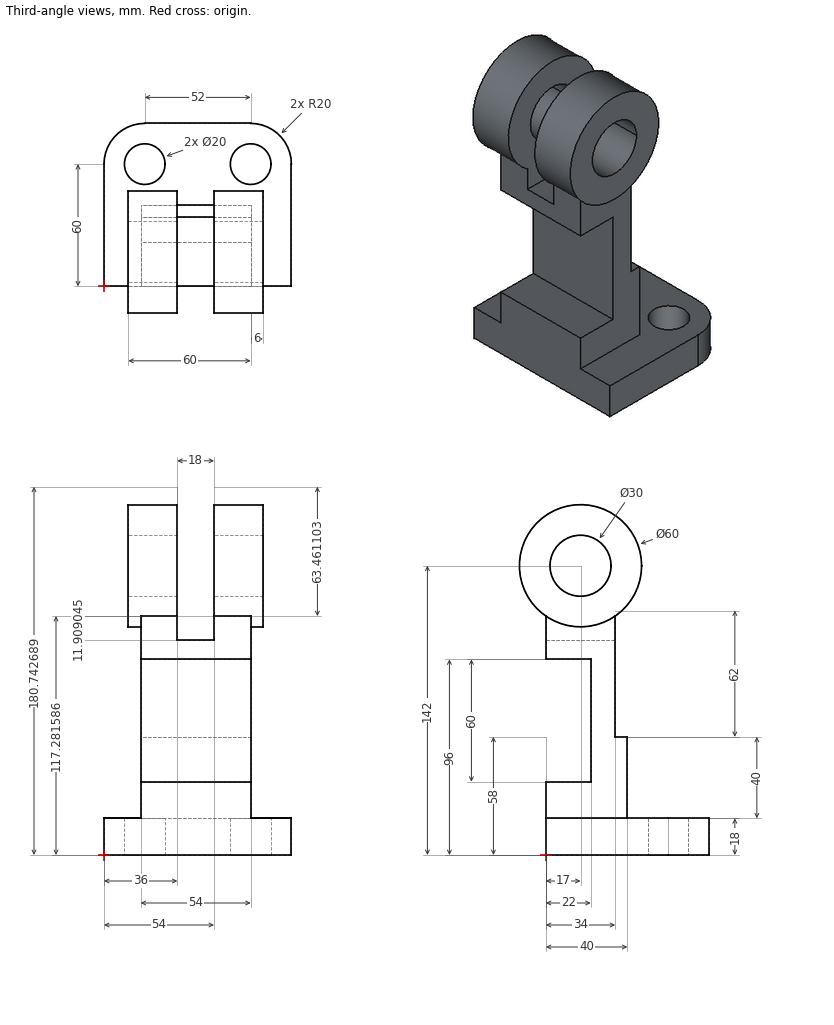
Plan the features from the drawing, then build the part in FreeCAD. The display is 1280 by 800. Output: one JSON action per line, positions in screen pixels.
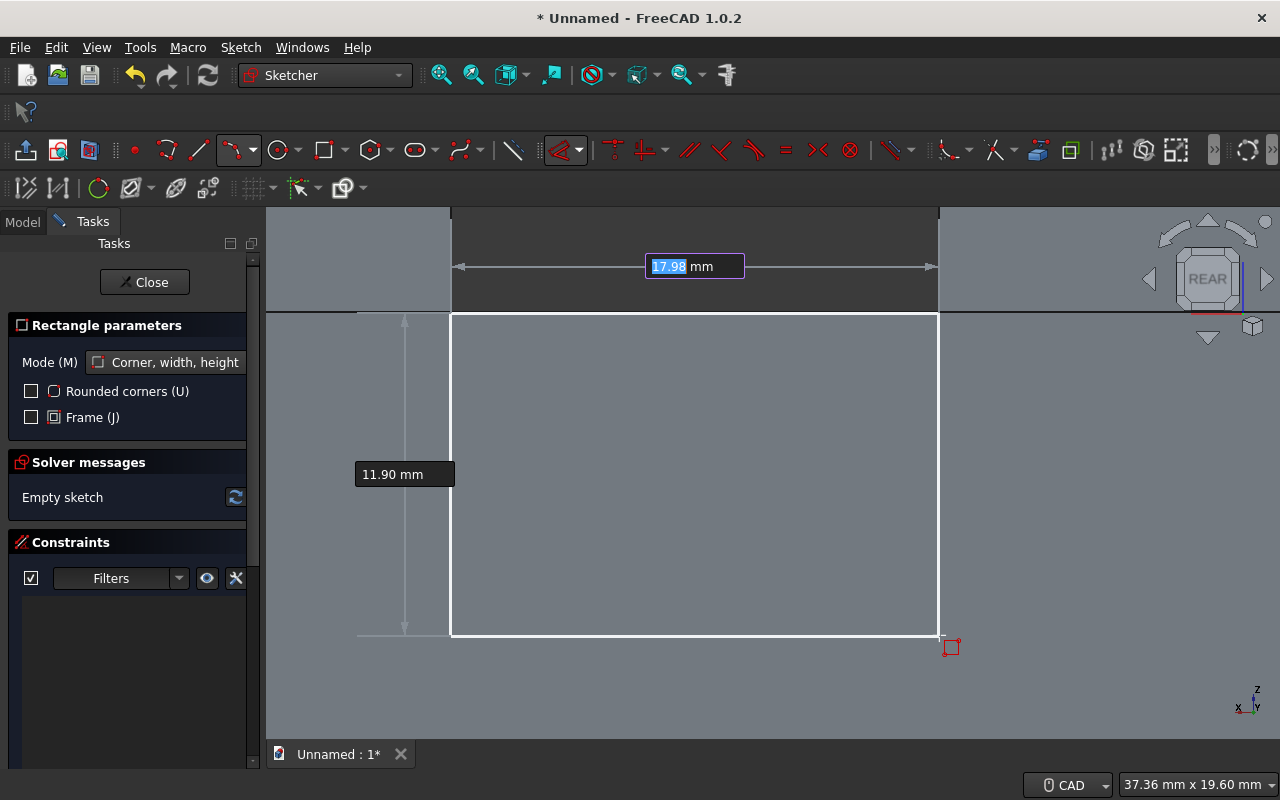
{"action": "type", "text": "18"}
{"action": "key", "text": "Tab"}
{"action": "type", "text": "11.909045"}
{"action": "key", "text": "Return"}
{"action": "key", "text": "Escape"}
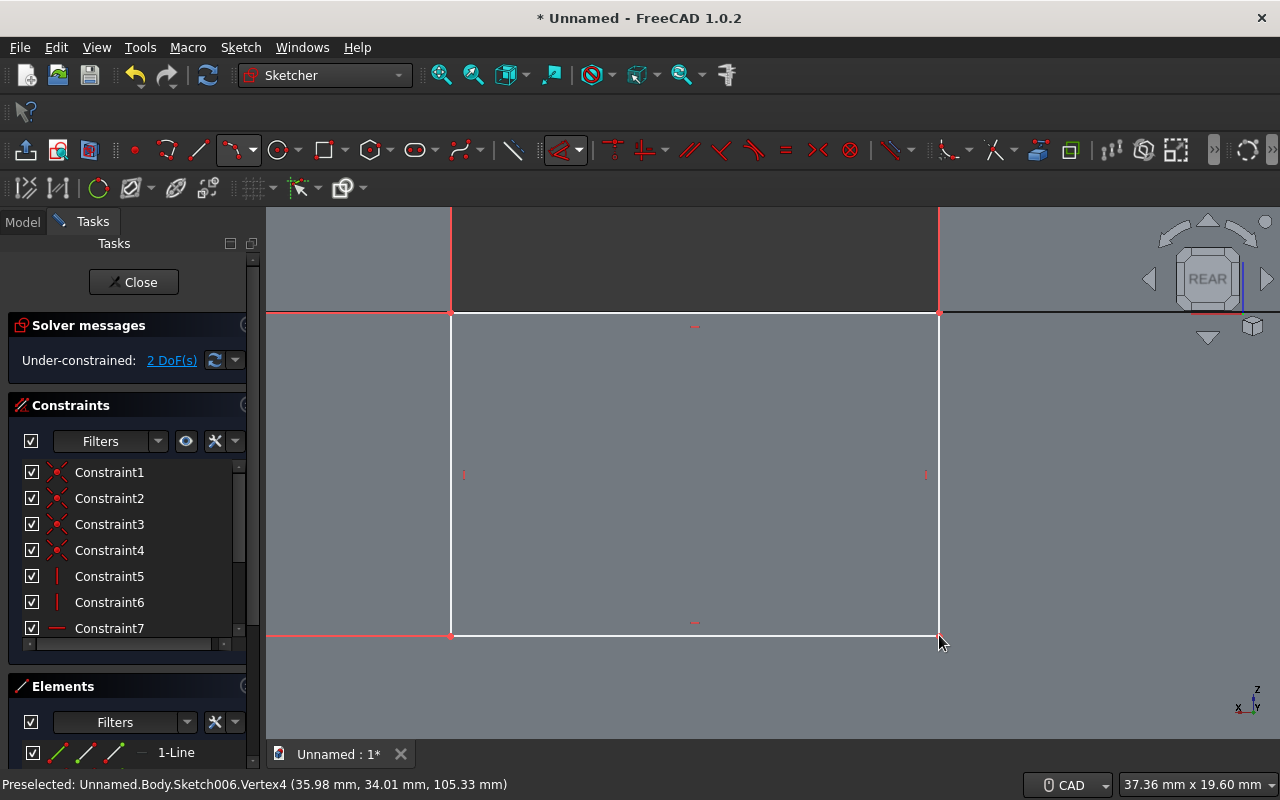
{"action": "left_click", "coordinate": [451, 313]}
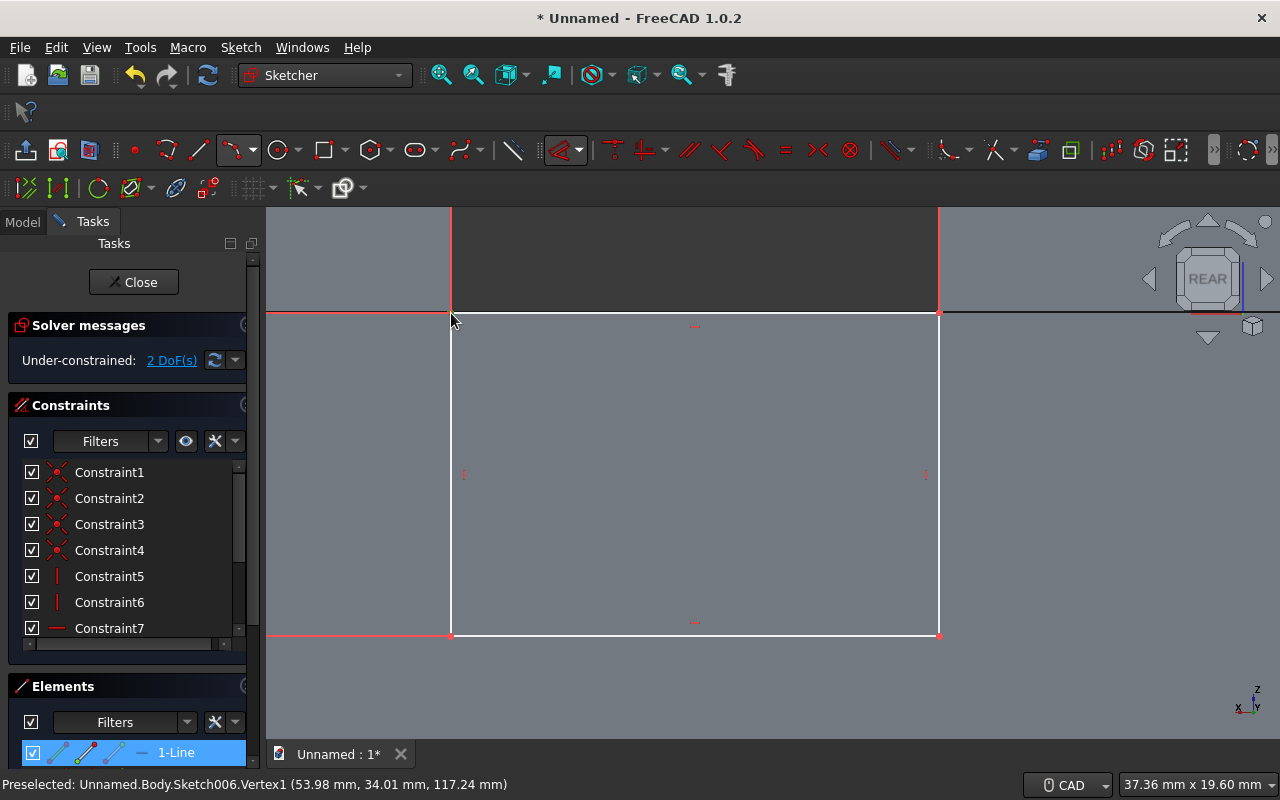
{"action": "left_click", "coordinate": [582, 150]}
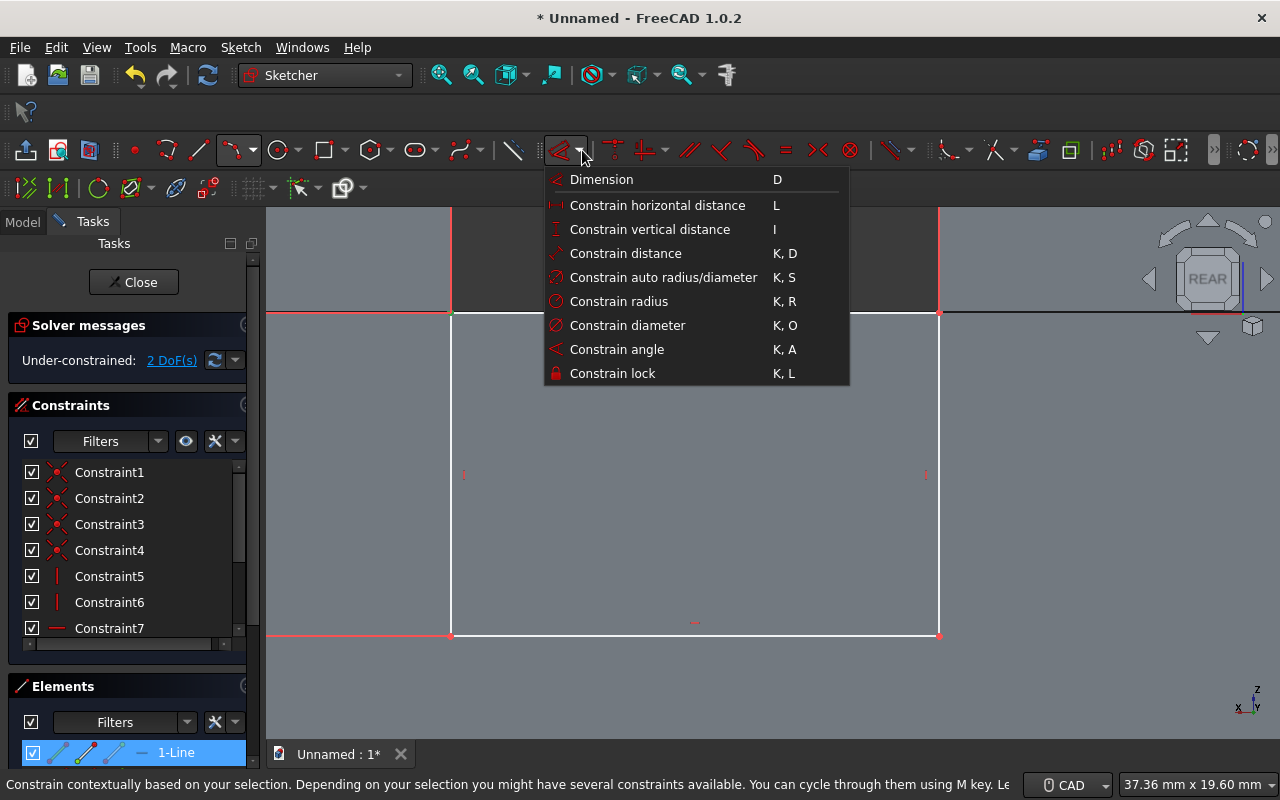
{"action": "left_click", "coordinate": [697, 205]}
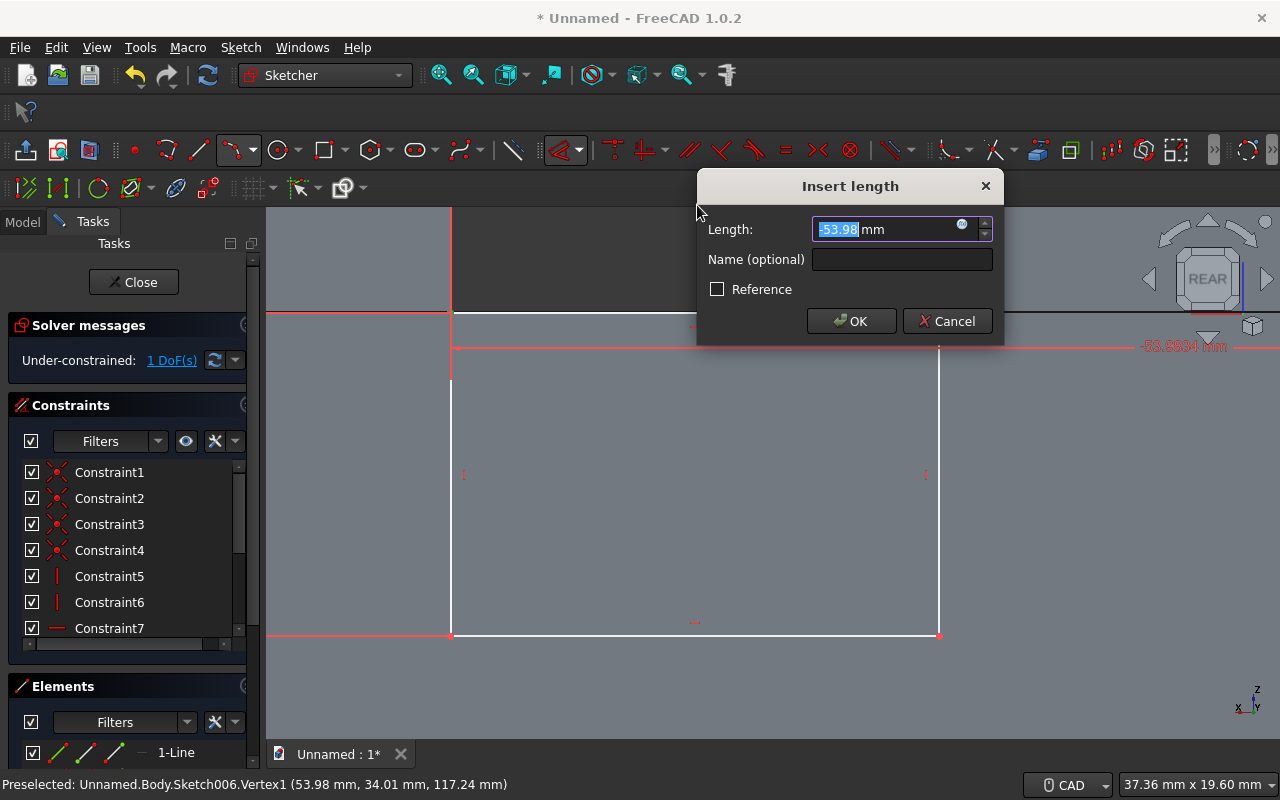
{"action": "type", "text": "-54"}
{"action": "key", "text": "Return"}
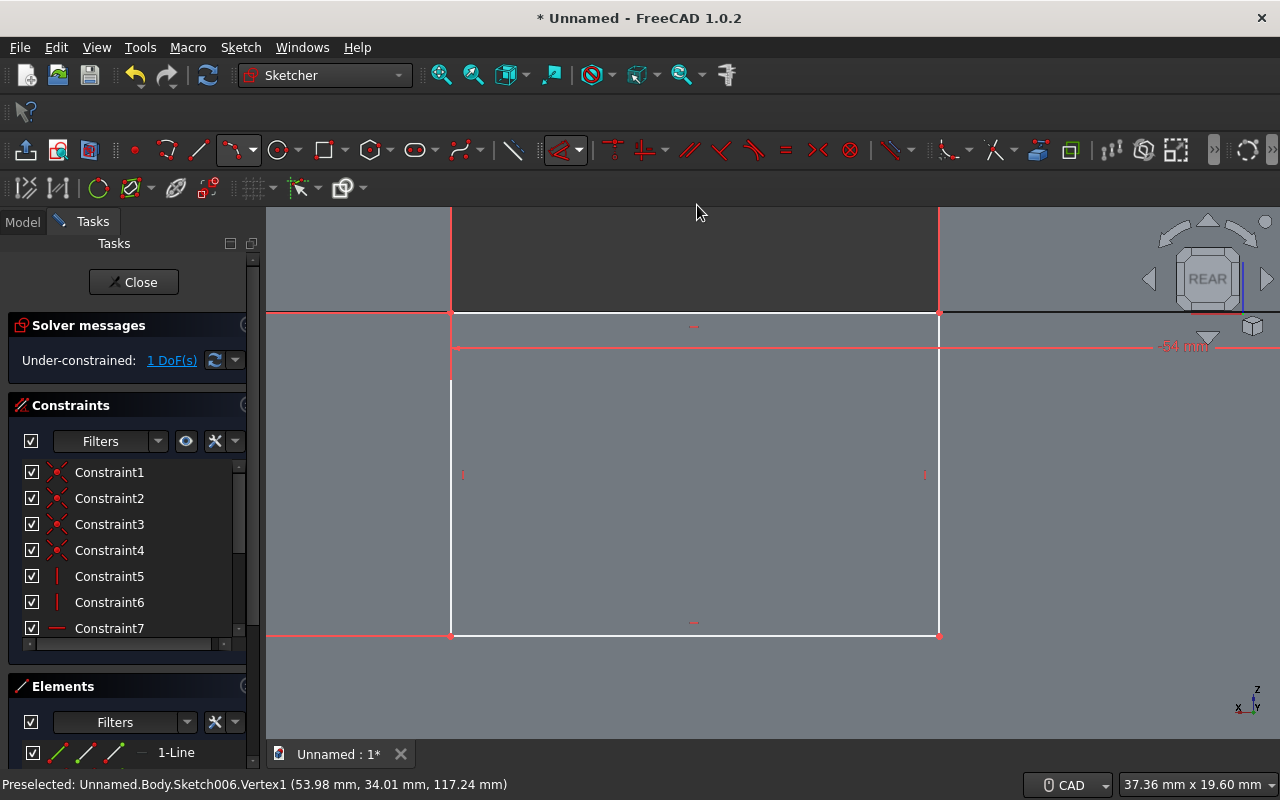
{"action": "left_click", "coordinate": [451, 313]}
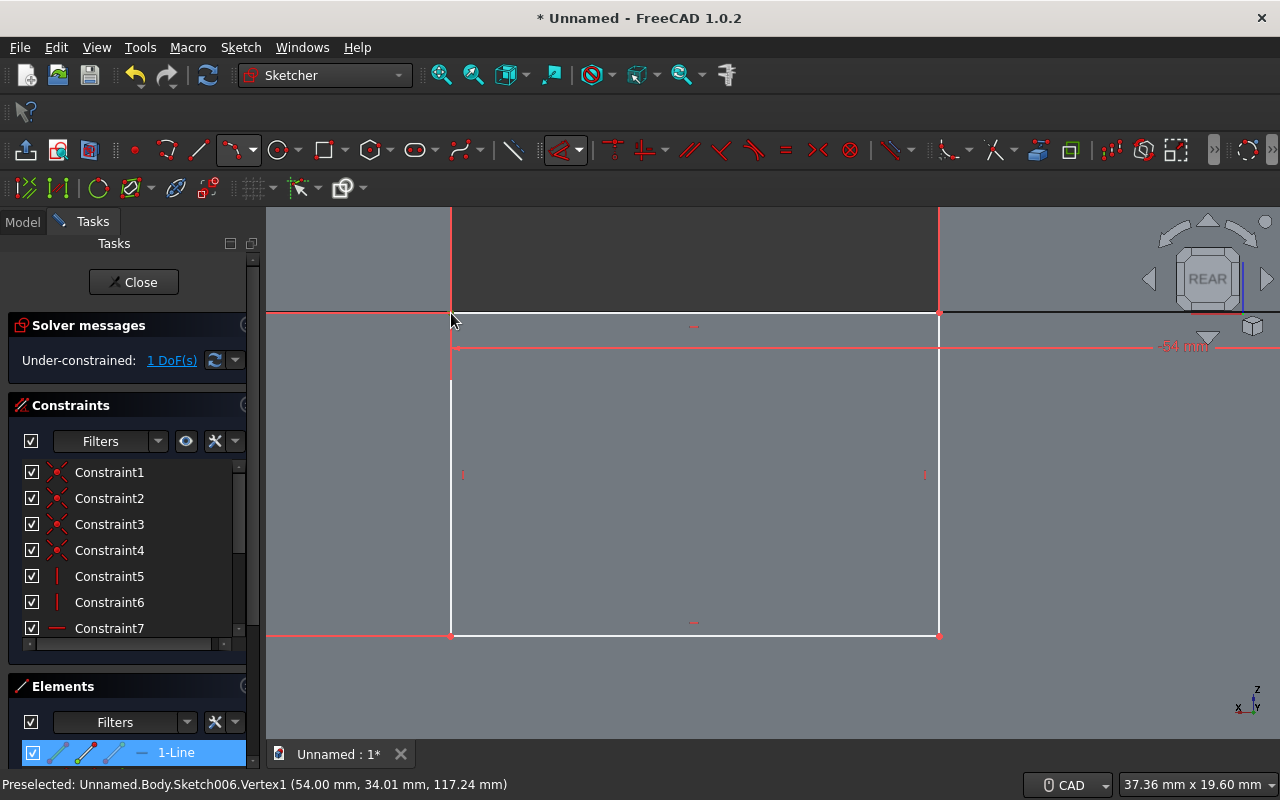
{"action": "left_click", "coordinate": [582, 150]}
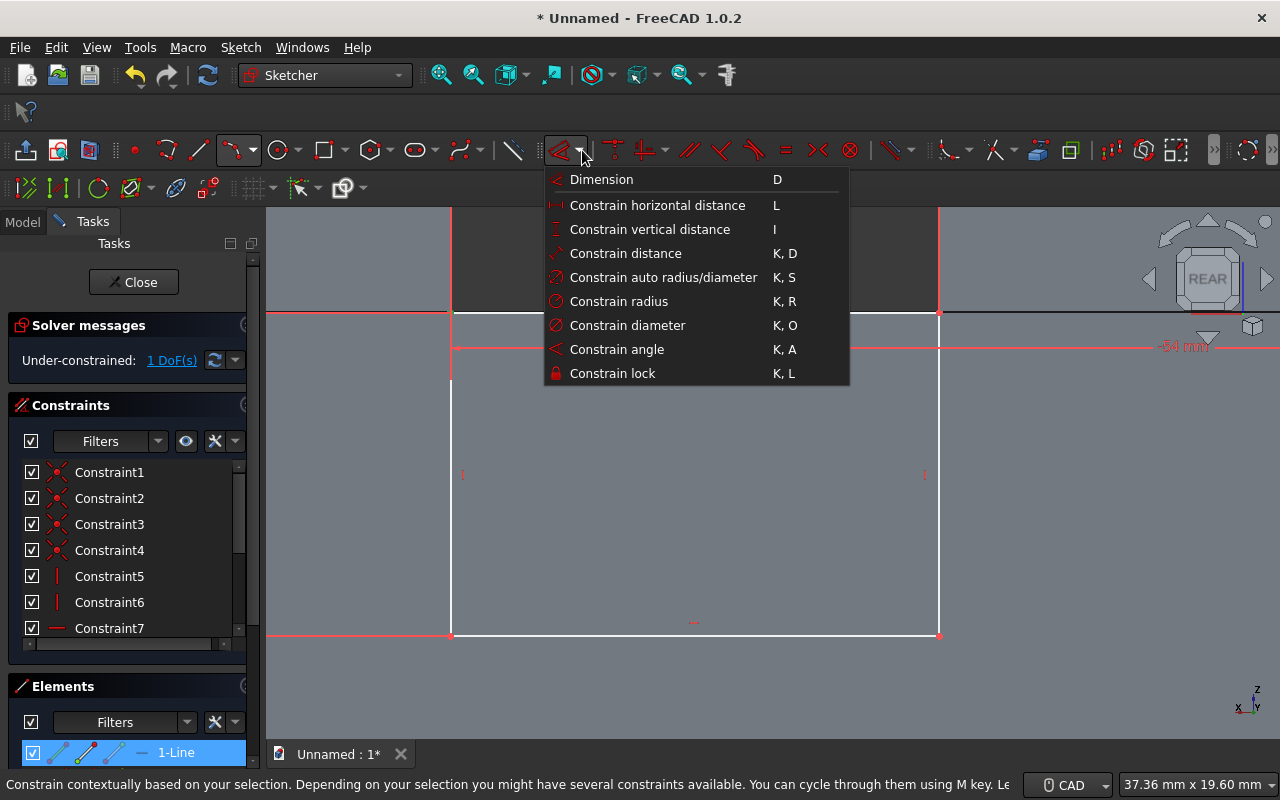
{"action": "left_click", "coordinate": [697, 229]}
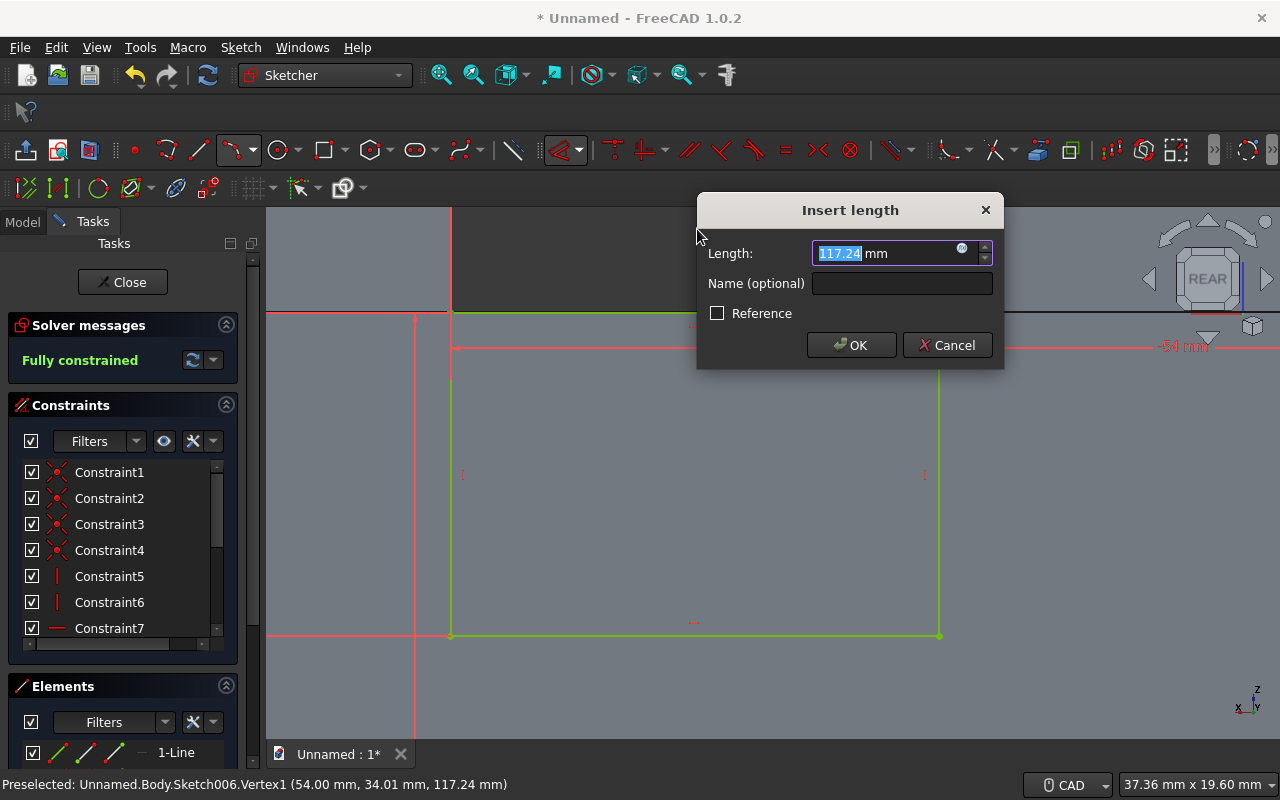
{"action": "type", "text": "117.281586"}
{"action": "key", "text": "Return"}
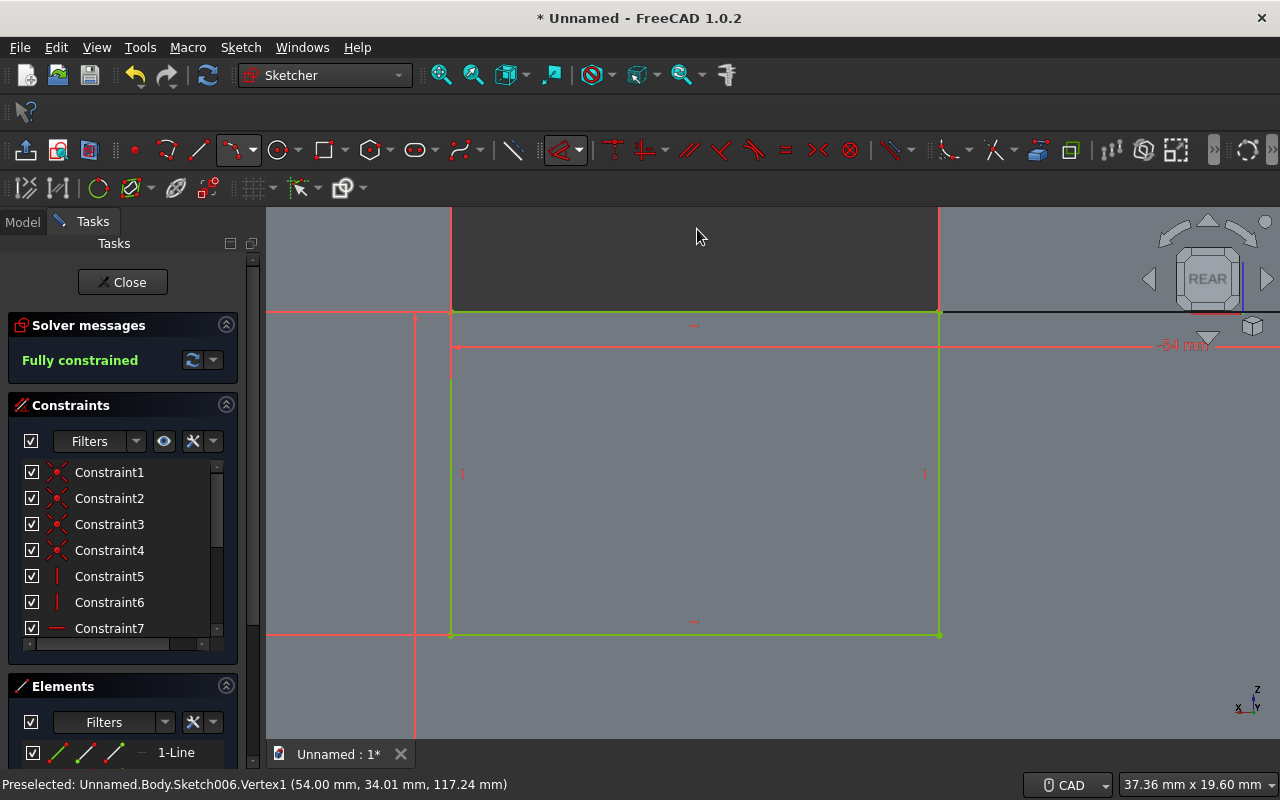
{"action": "left_click", "coordinate": [123, 282]}